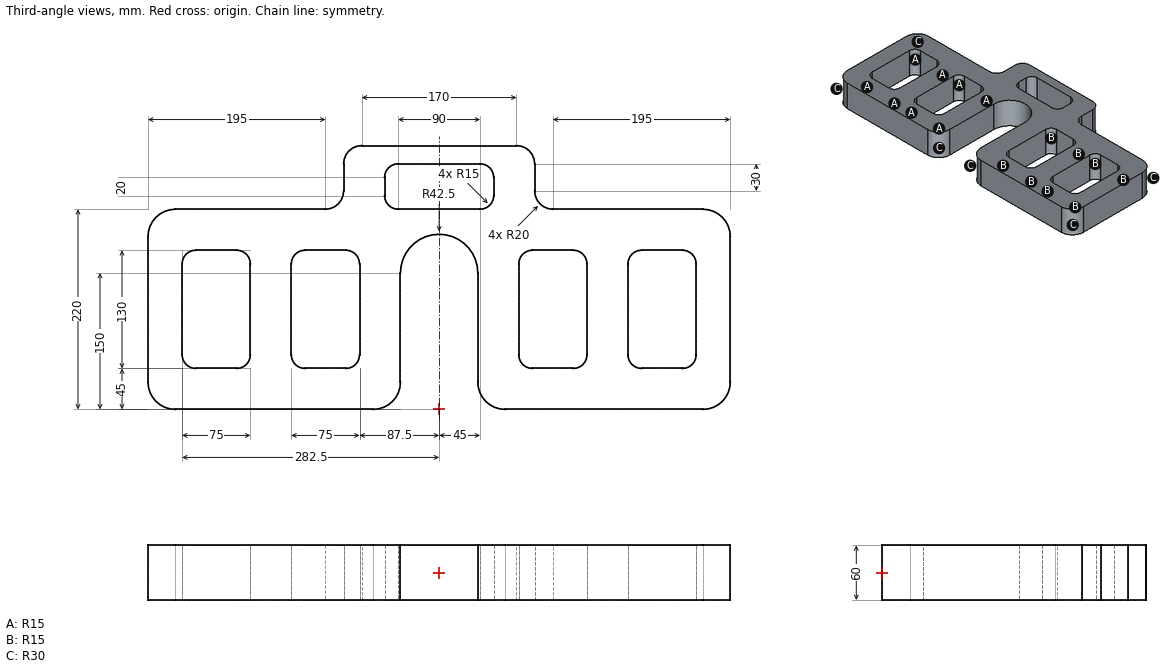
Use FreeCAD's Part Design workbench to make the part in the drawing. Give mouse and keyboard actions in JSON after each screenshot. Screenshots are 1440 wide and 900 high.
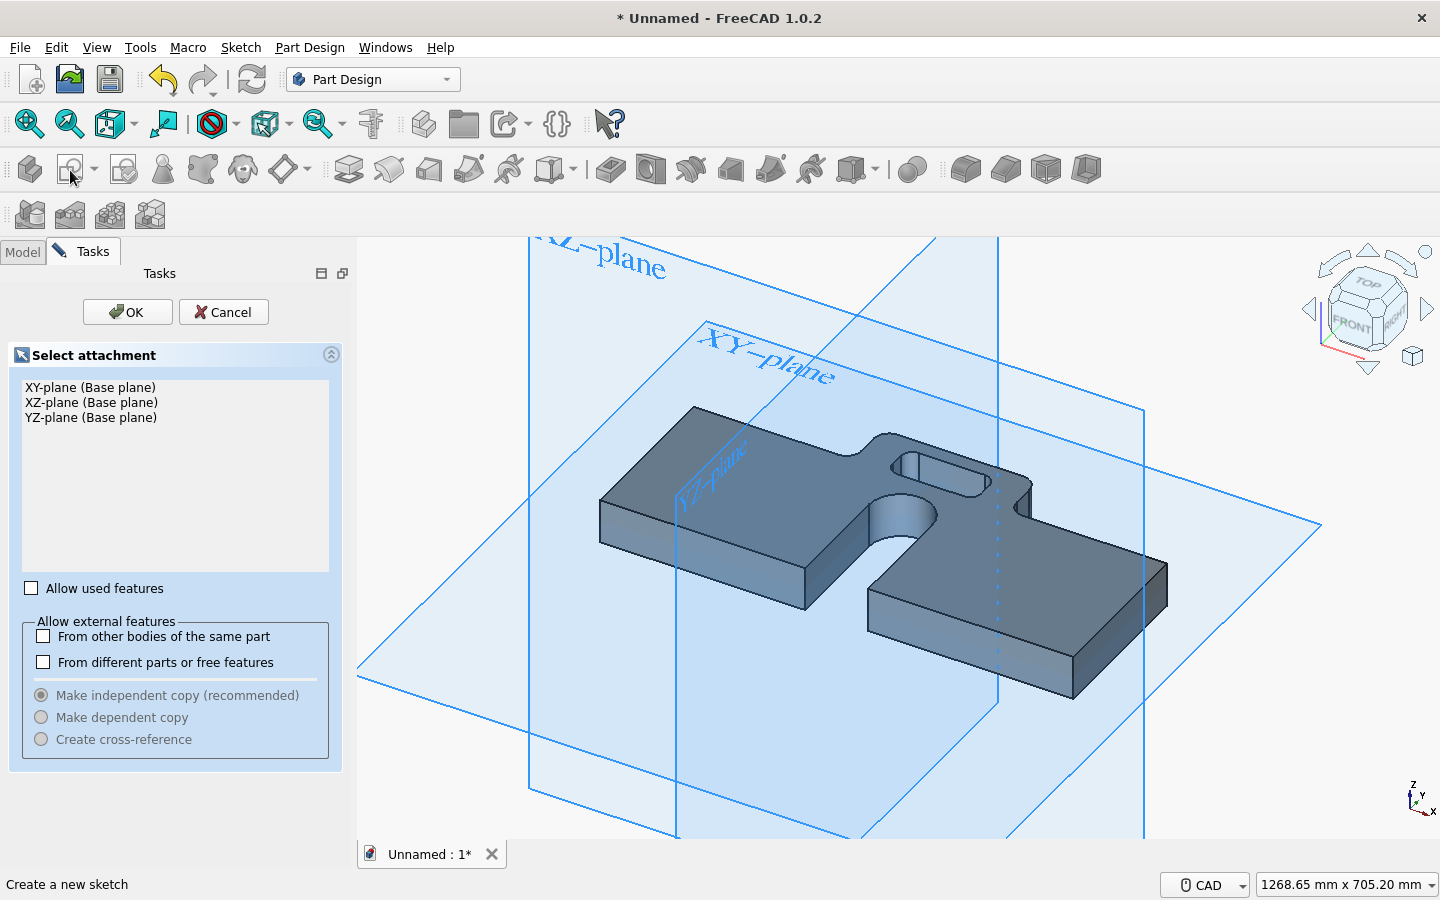
{"action": "left_click", "coordinate": [82, 388]}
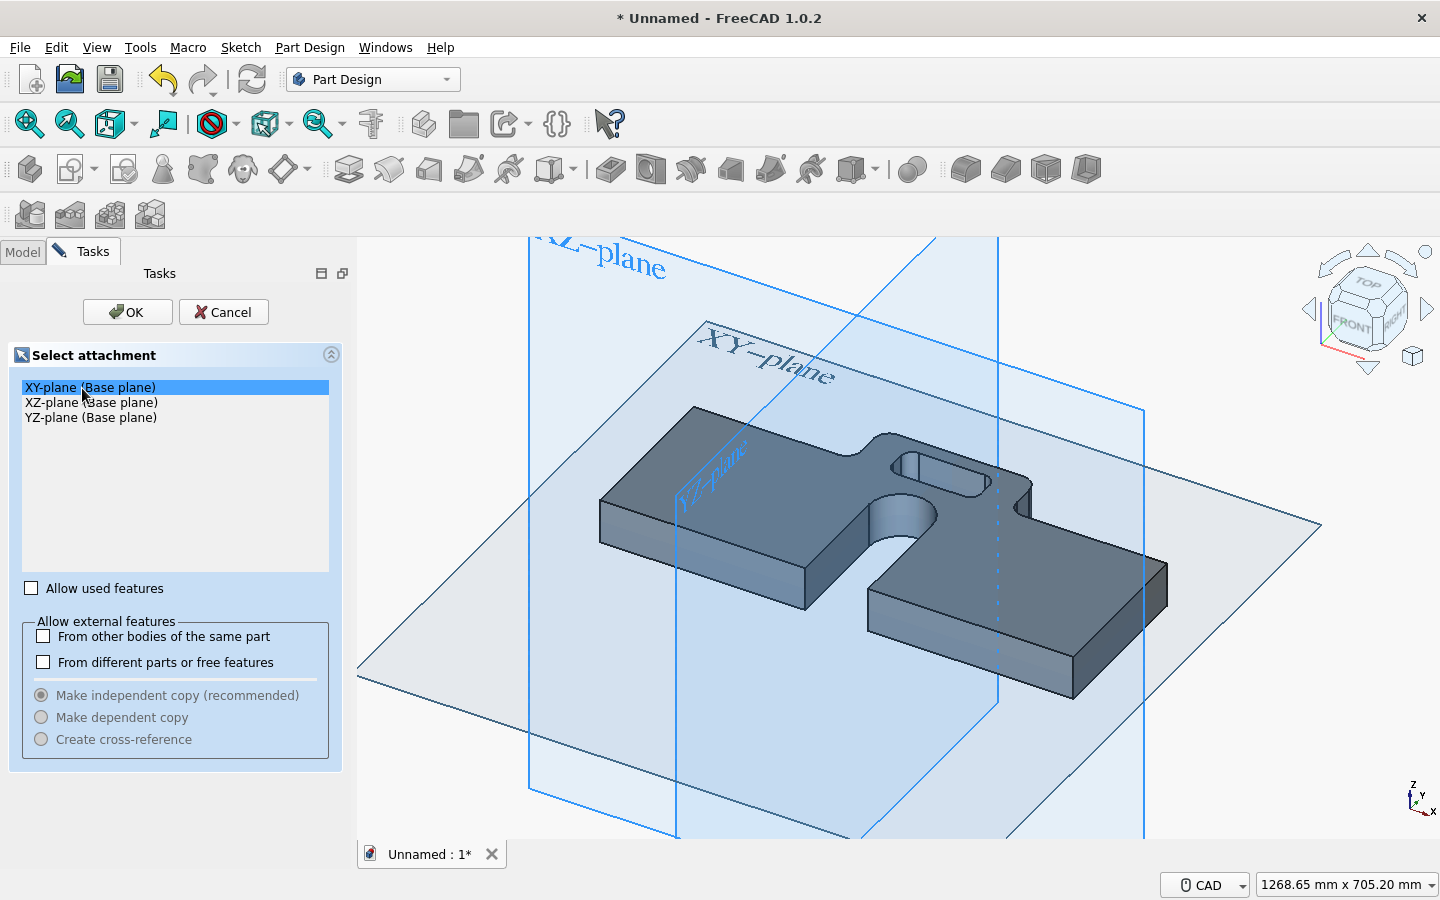
{"action": "left_click", "coordinate": [128, 312]}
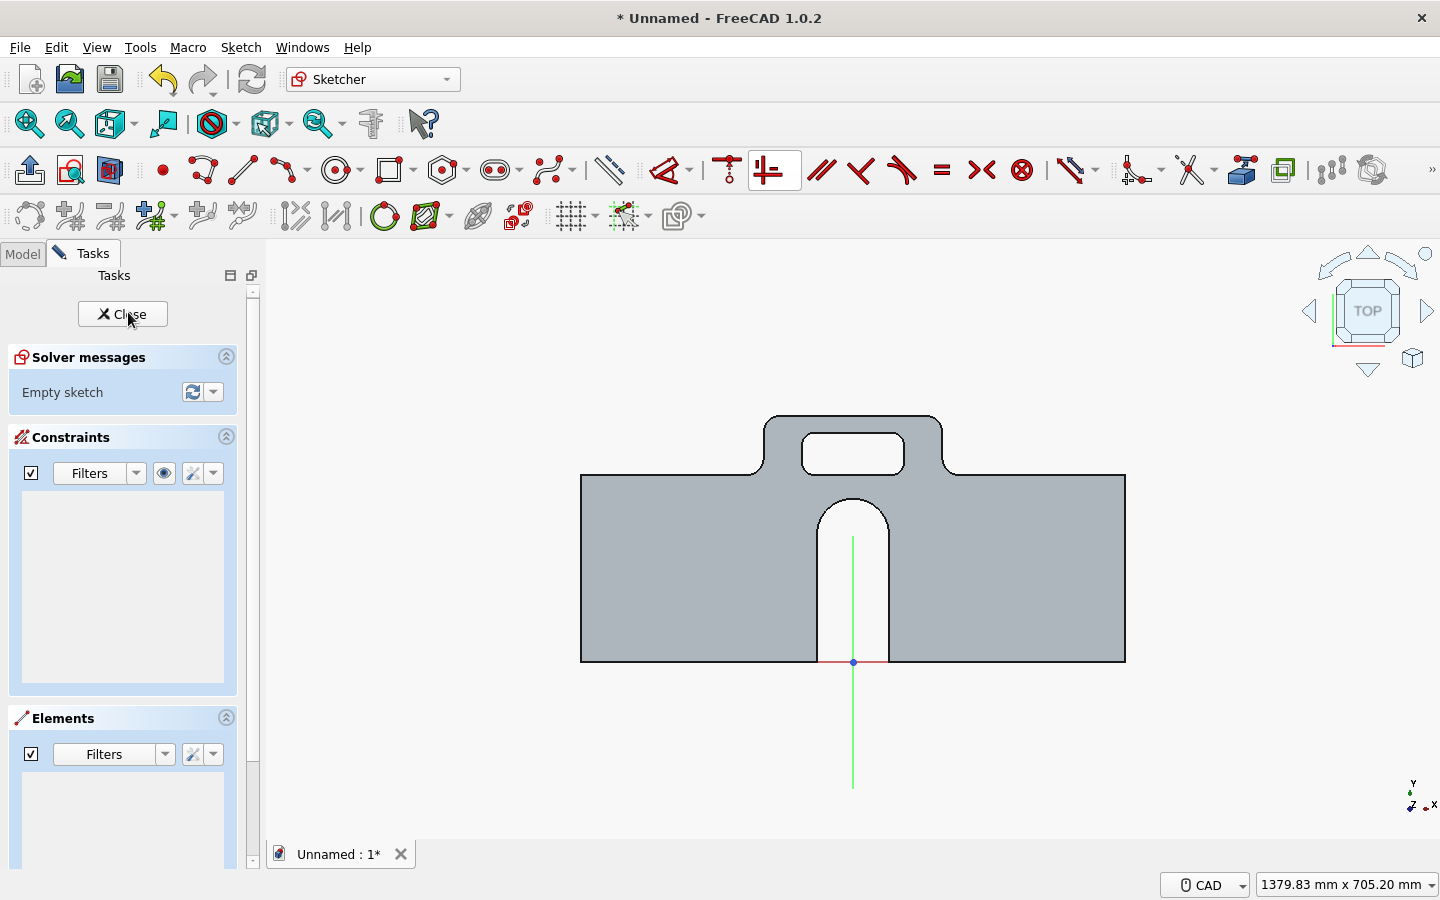
{"action": "left_click", "coordinate": [110, 170]}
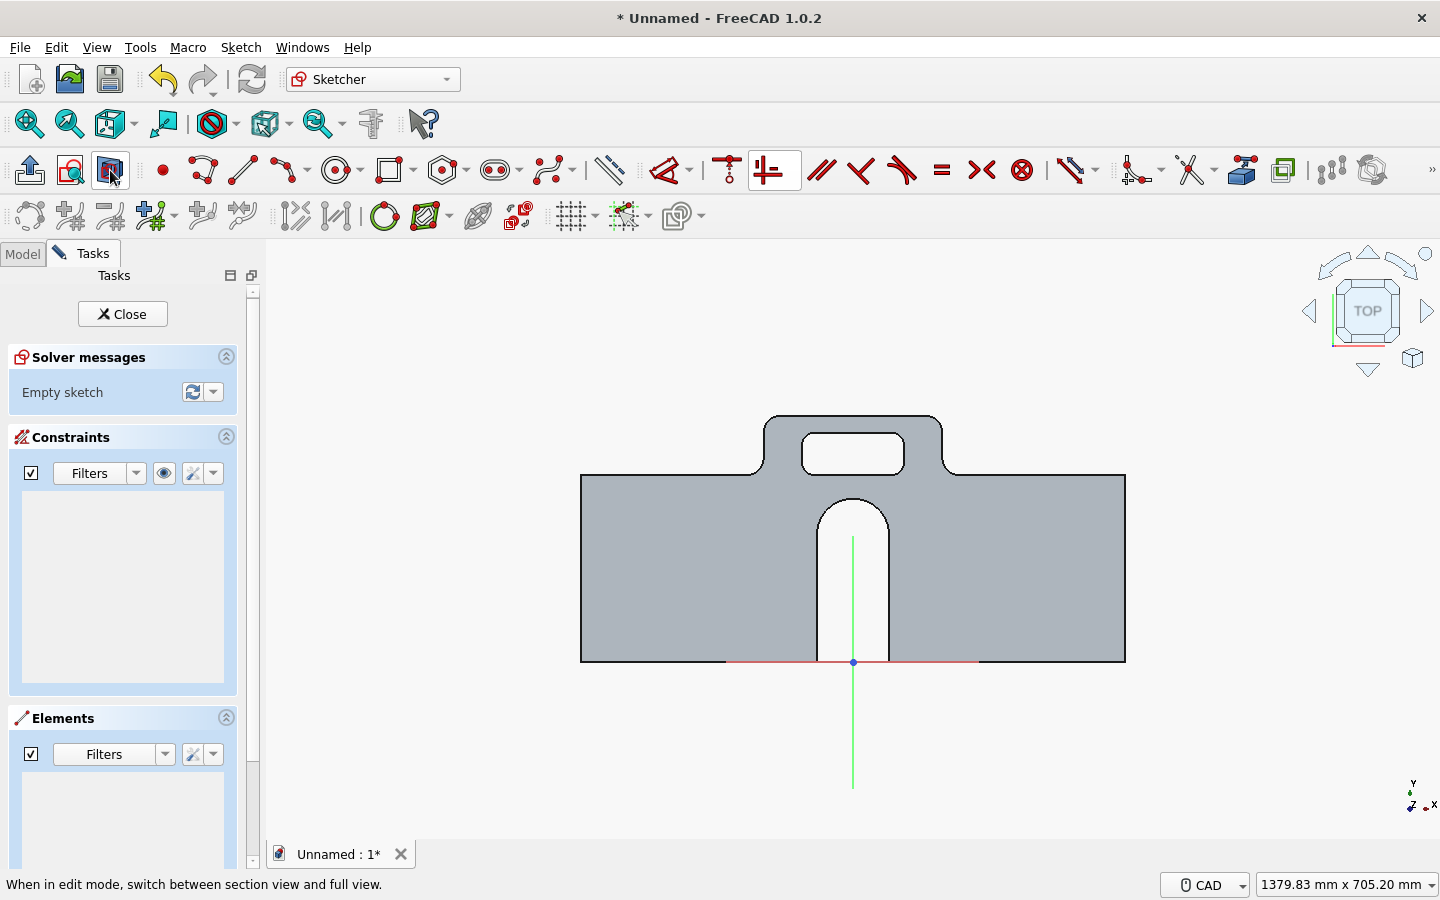
{"action": "scroll", "coordinate": [703, 616], "scroll_direction": "up", "scroll_amount": 5}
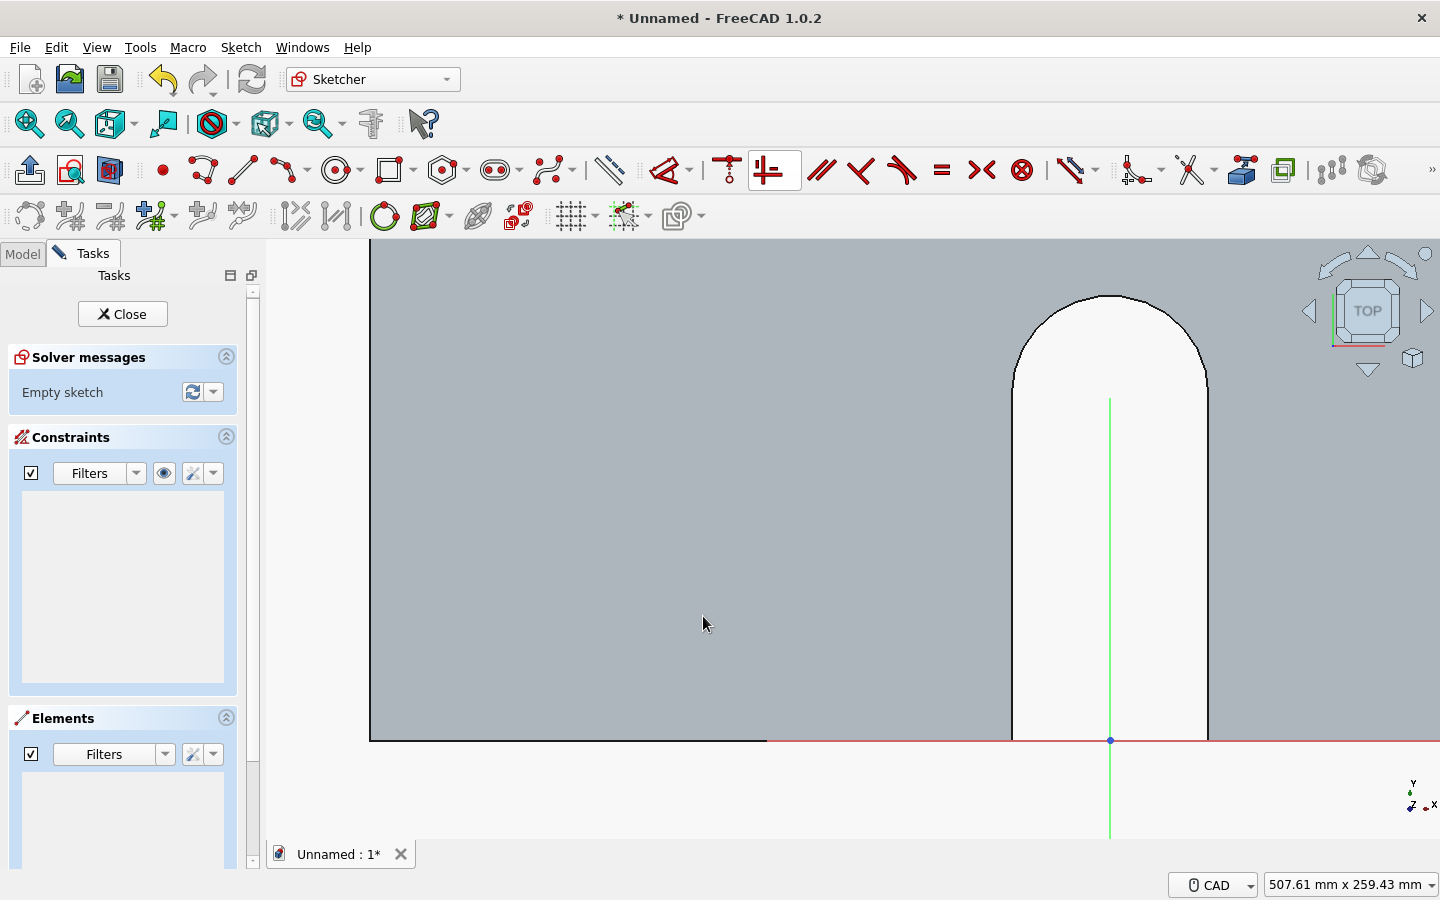
{"action": "key", "text": "g r"}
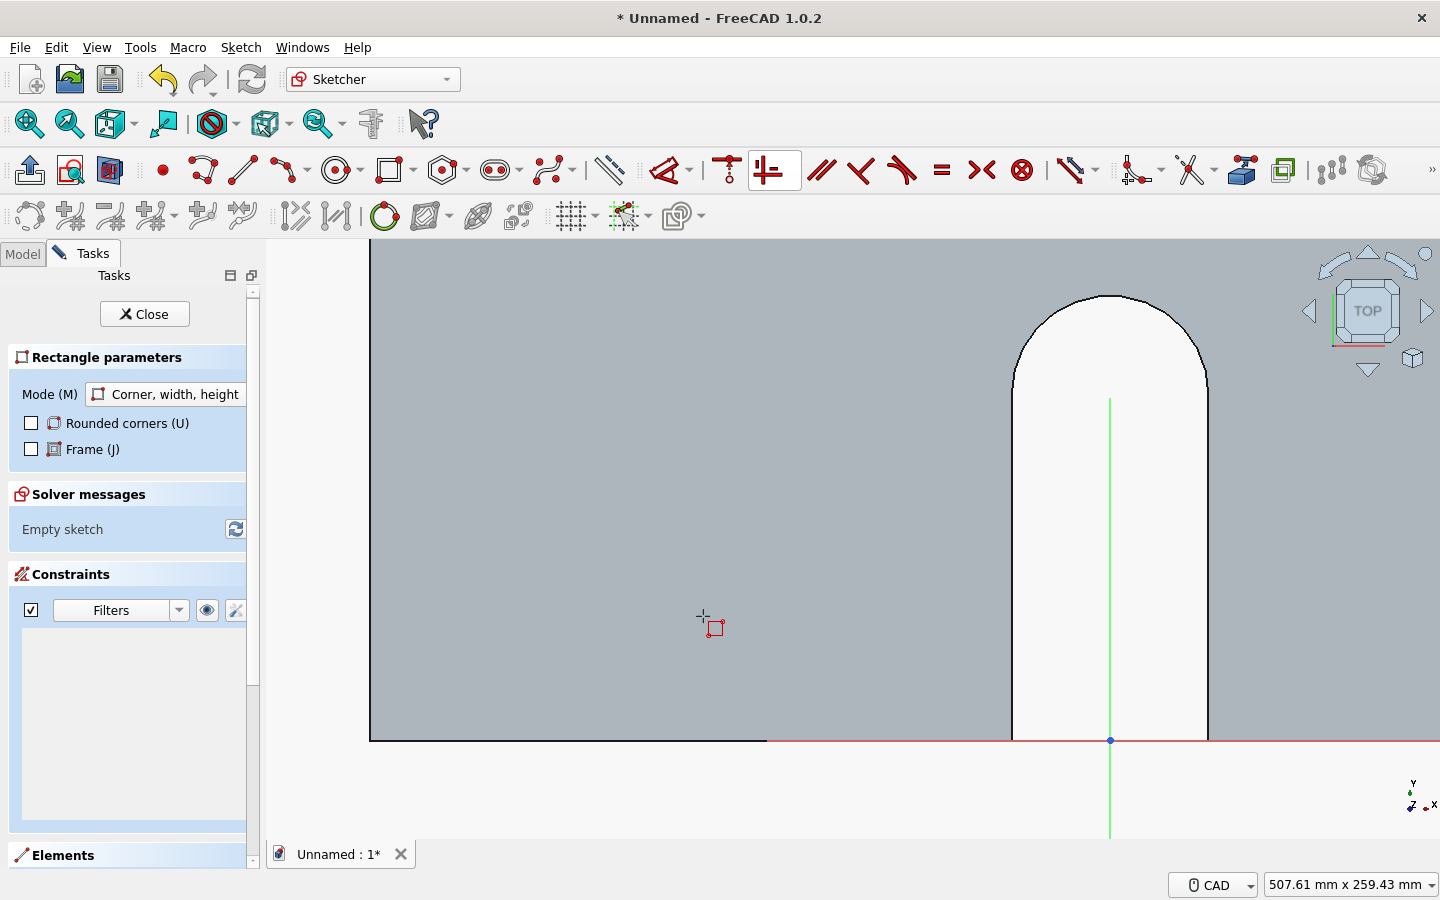
{"action": "left_click", "coordinate": [457, 336]}
{"action": "mouse_move", "coordinate": [630, 637]}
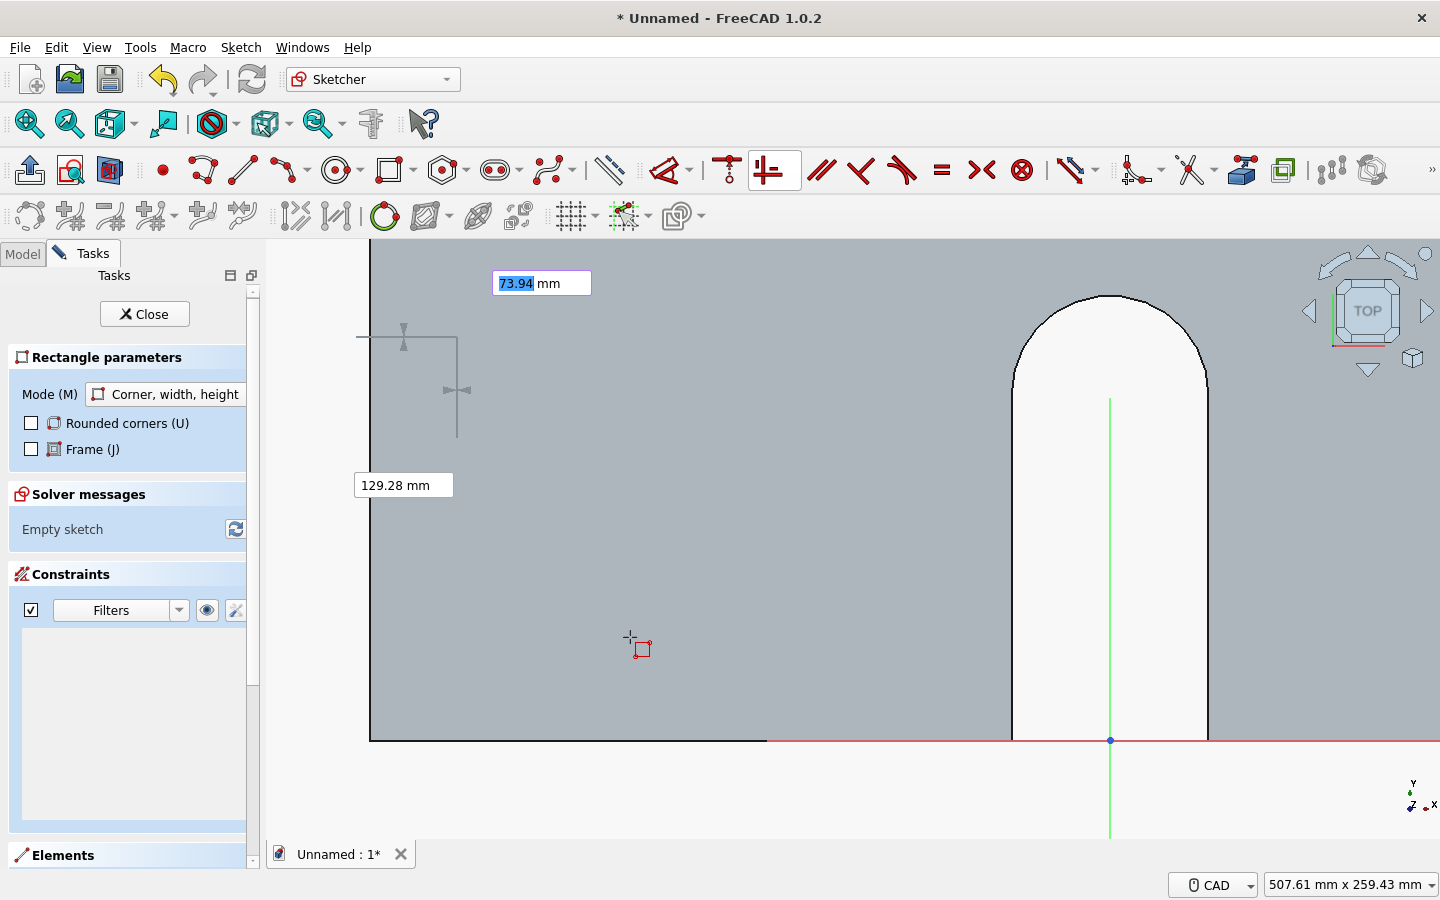
{"action": "type", "text": "75"}
{"action": "key", "text": "Tab"}
{"action": "type", "text": "130"}
{"action": "key", "text": "Return"}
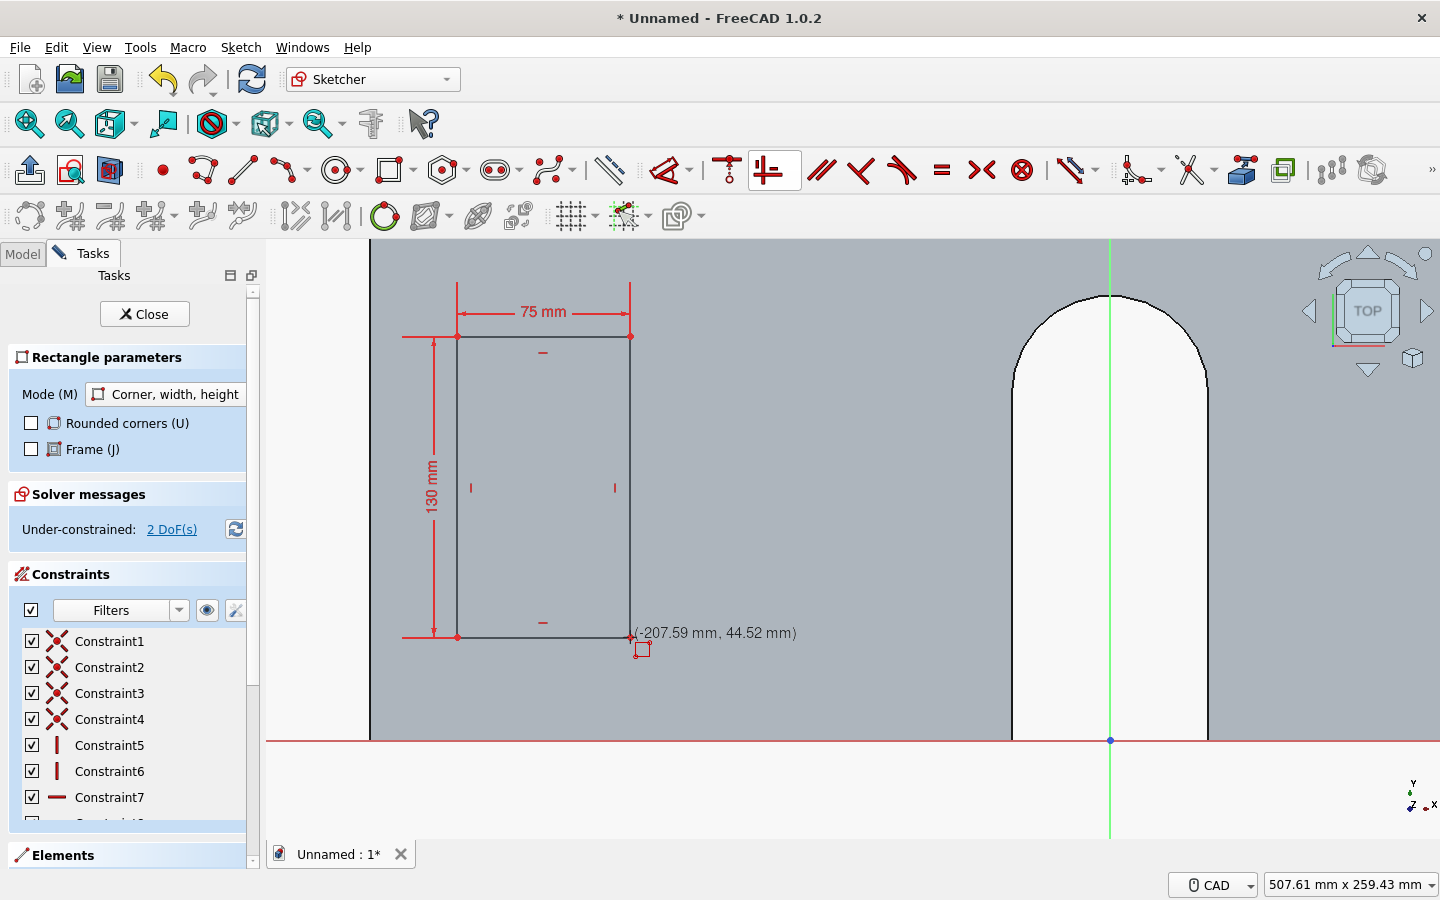
{"action": "left_click", "coordinate": [734, 336]}
{"action": "mouse_move", "coordinate": [908, 637]}